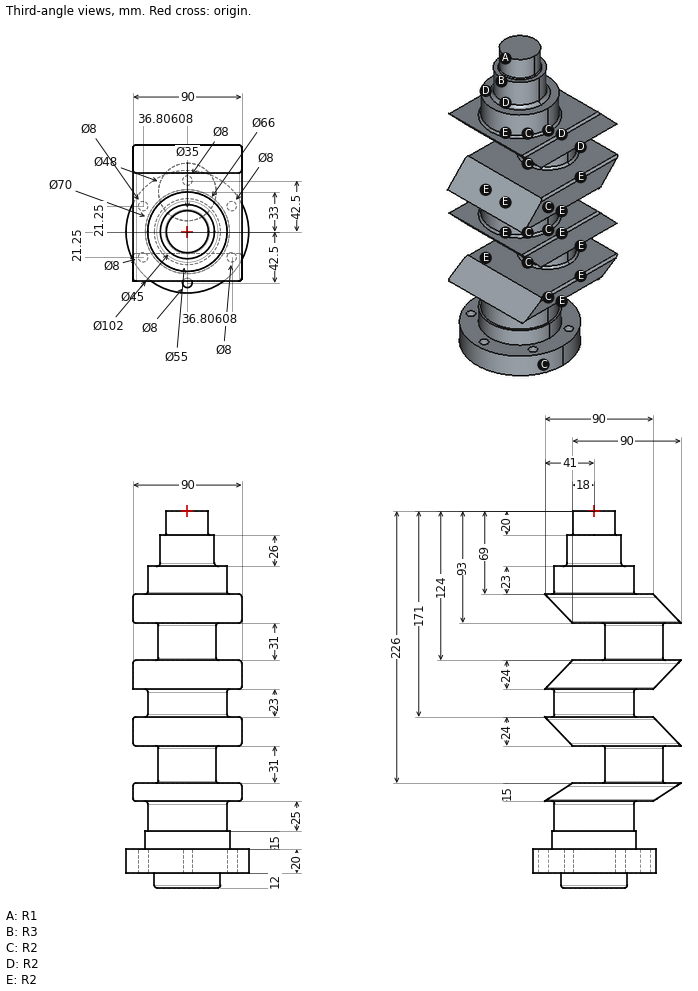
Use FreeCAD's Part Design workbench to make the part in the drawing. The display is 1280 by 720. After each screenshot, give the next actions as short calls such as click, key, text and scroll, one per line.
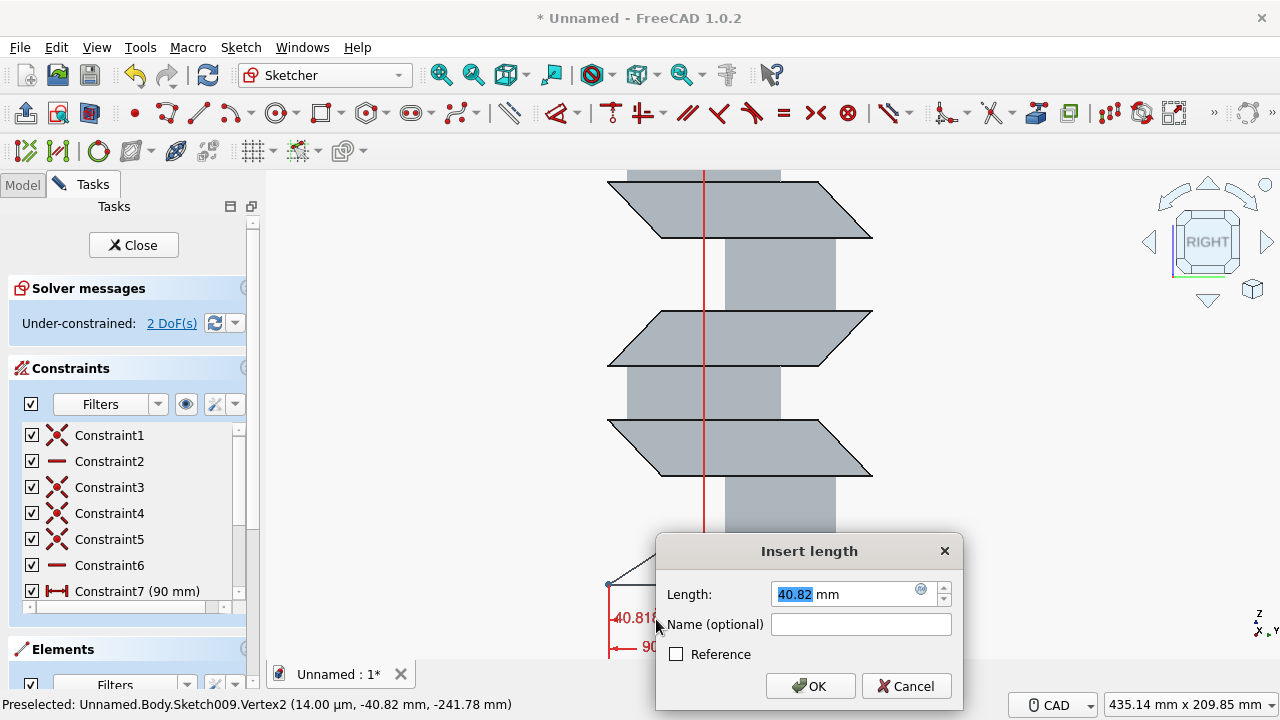
text(41)
key(Return)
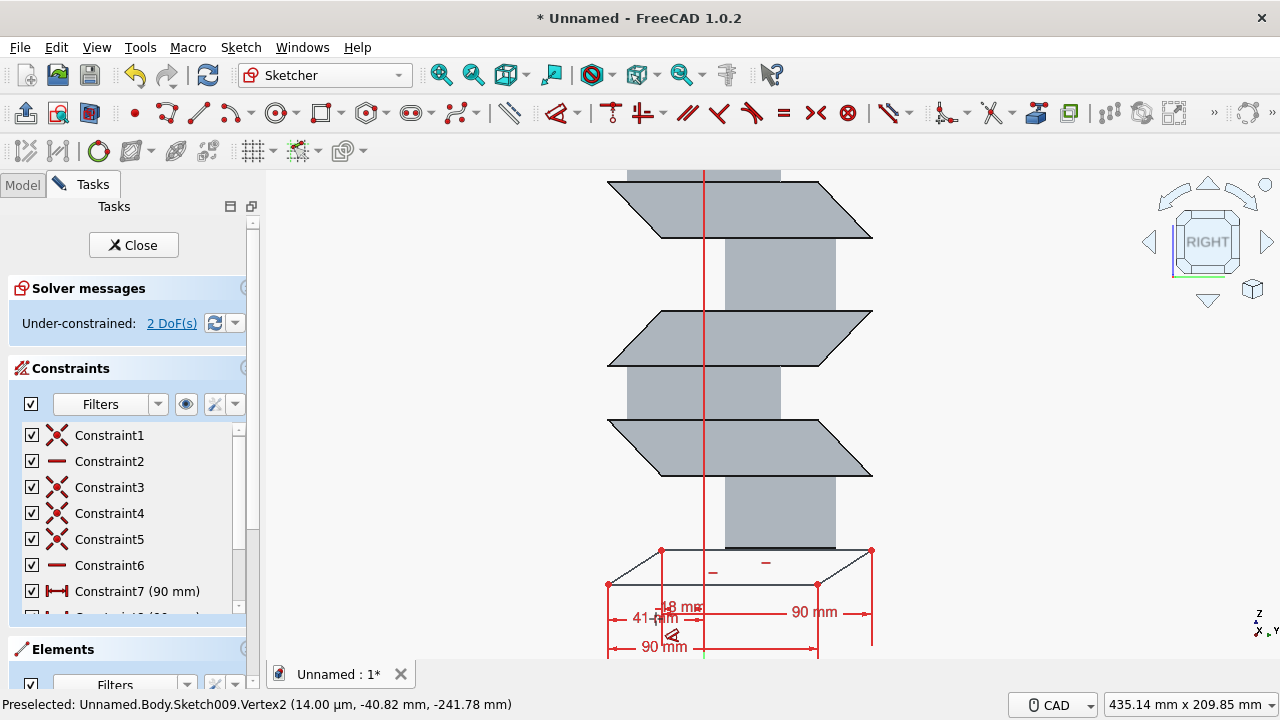
click(646, 561)
click(574, 568)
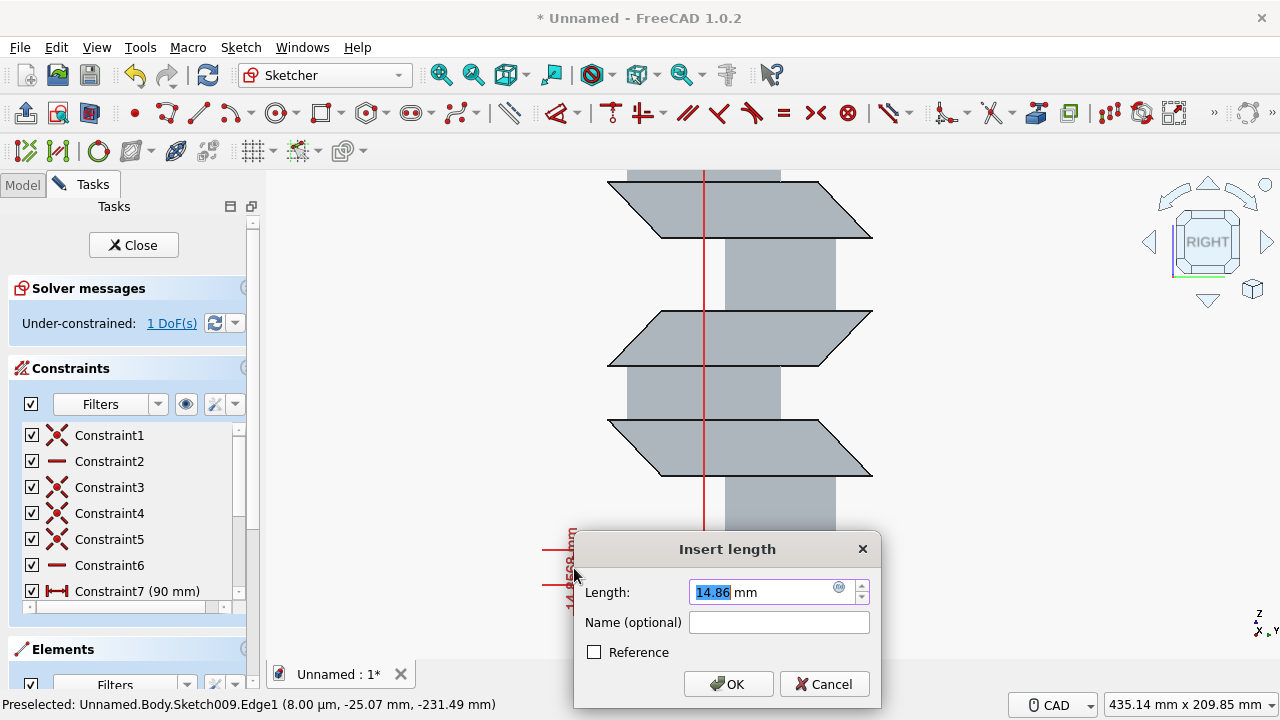
text(15)
key(Return)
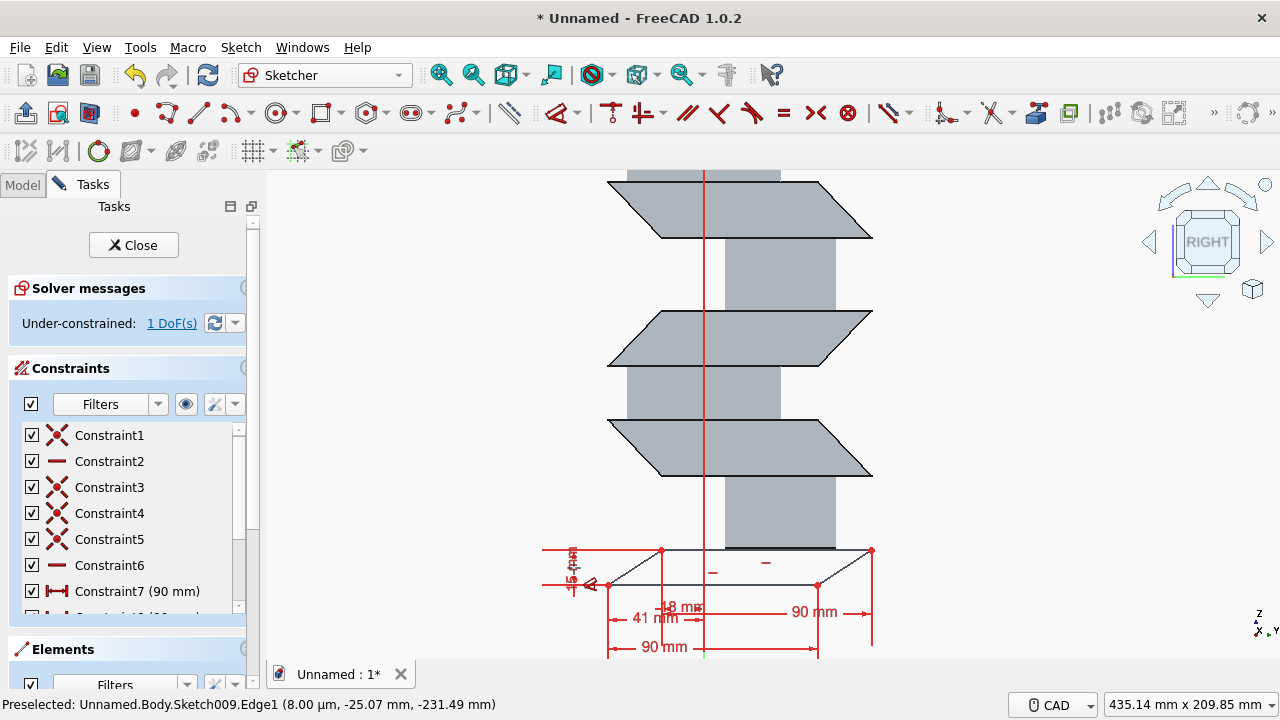
click(662, 550)
click(628, 374)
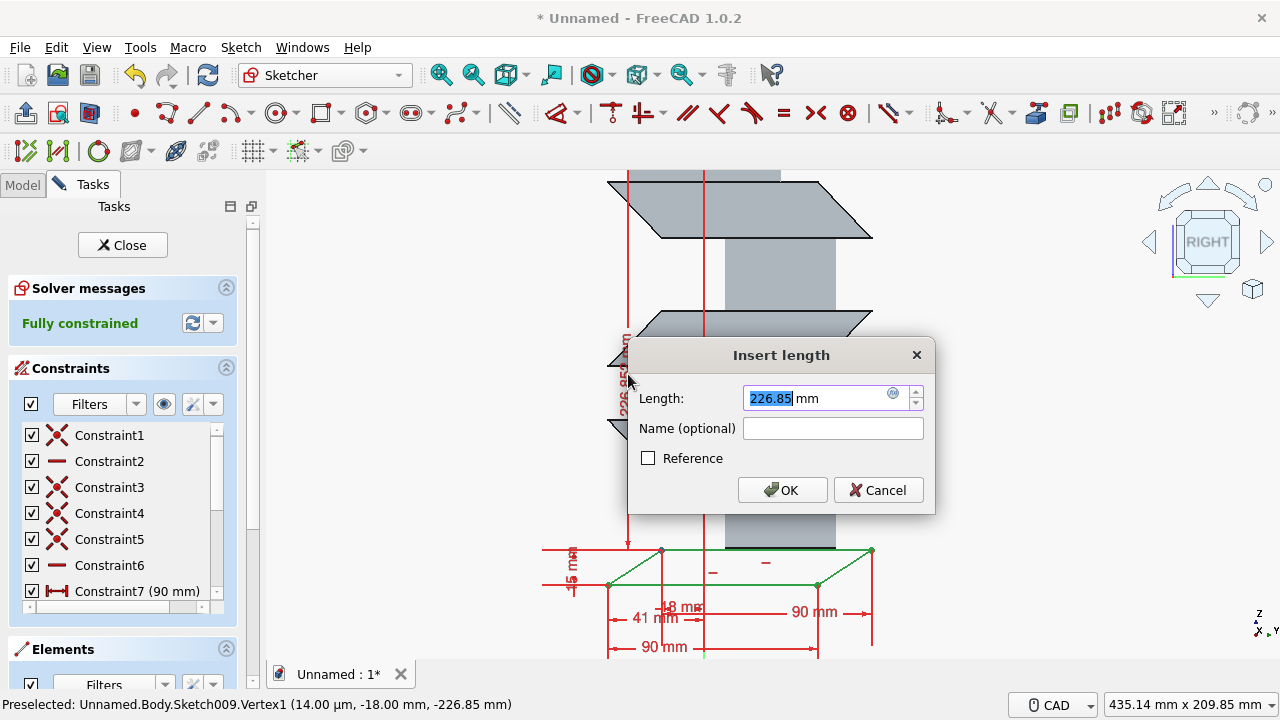
text(226)
key(Return)
key(Escape)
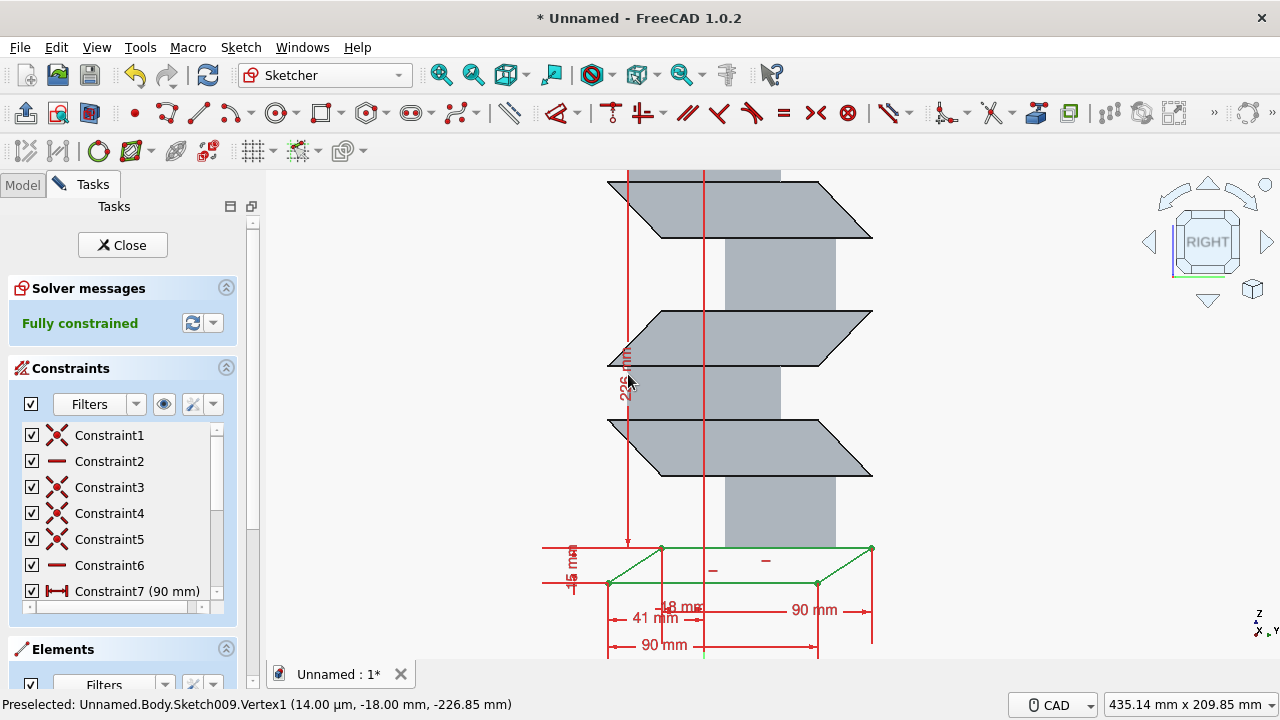
click(123, 245)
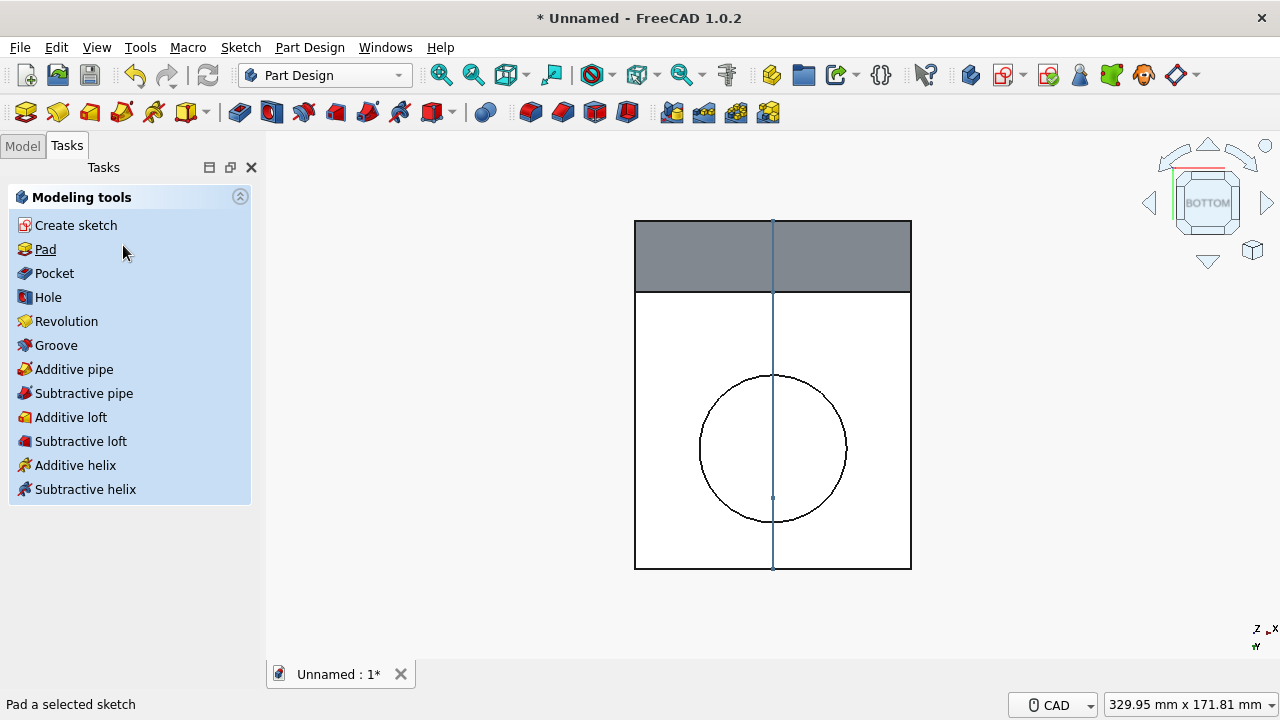
click(26, 112)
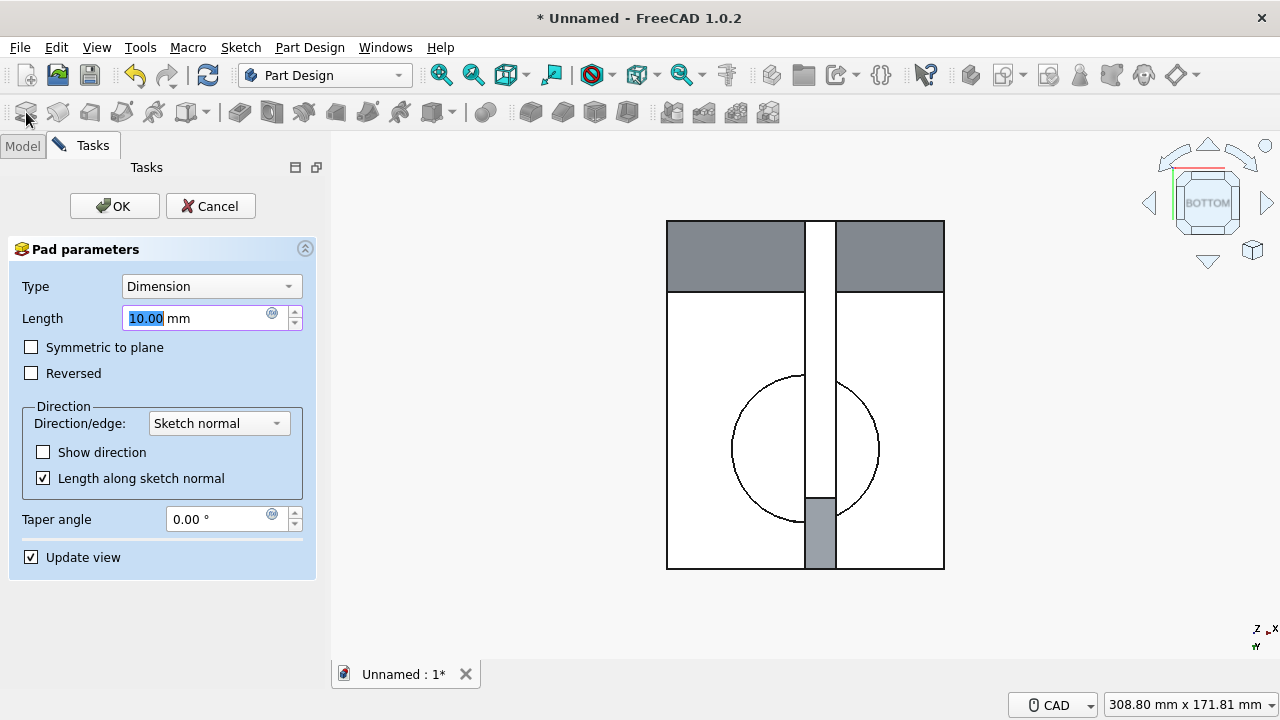
text(90)
key(Tab)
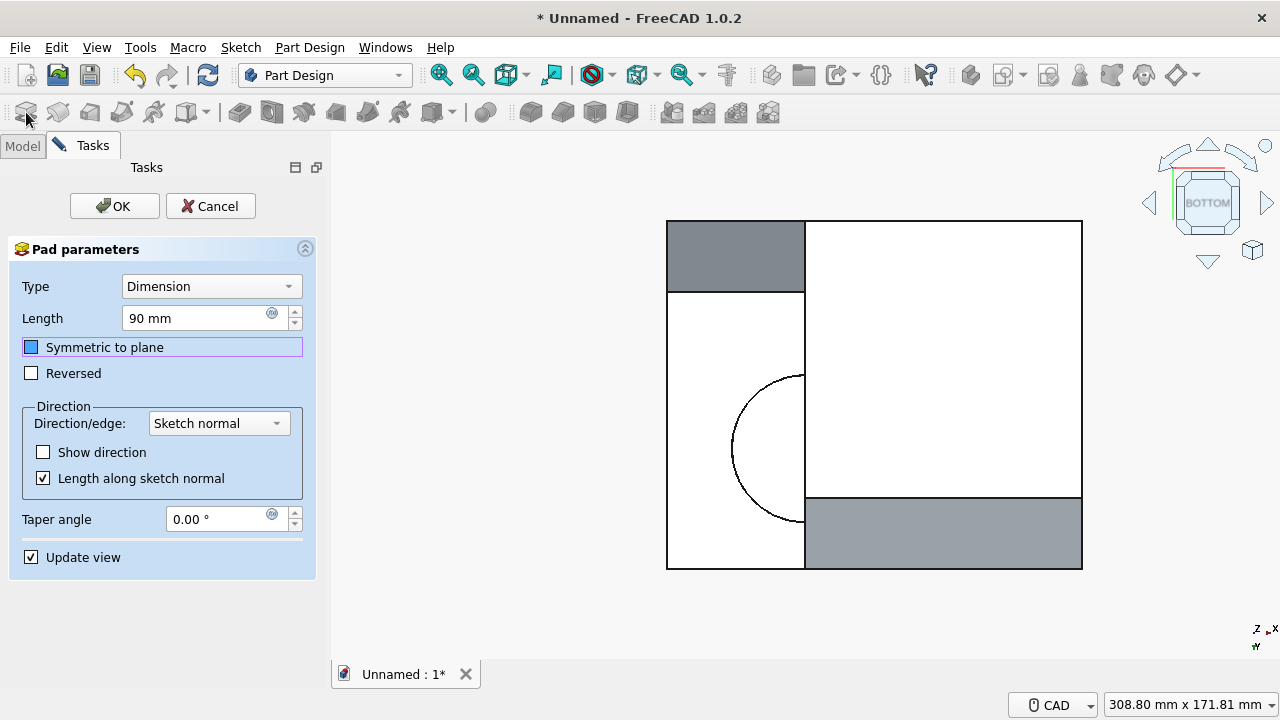
click(30, 347)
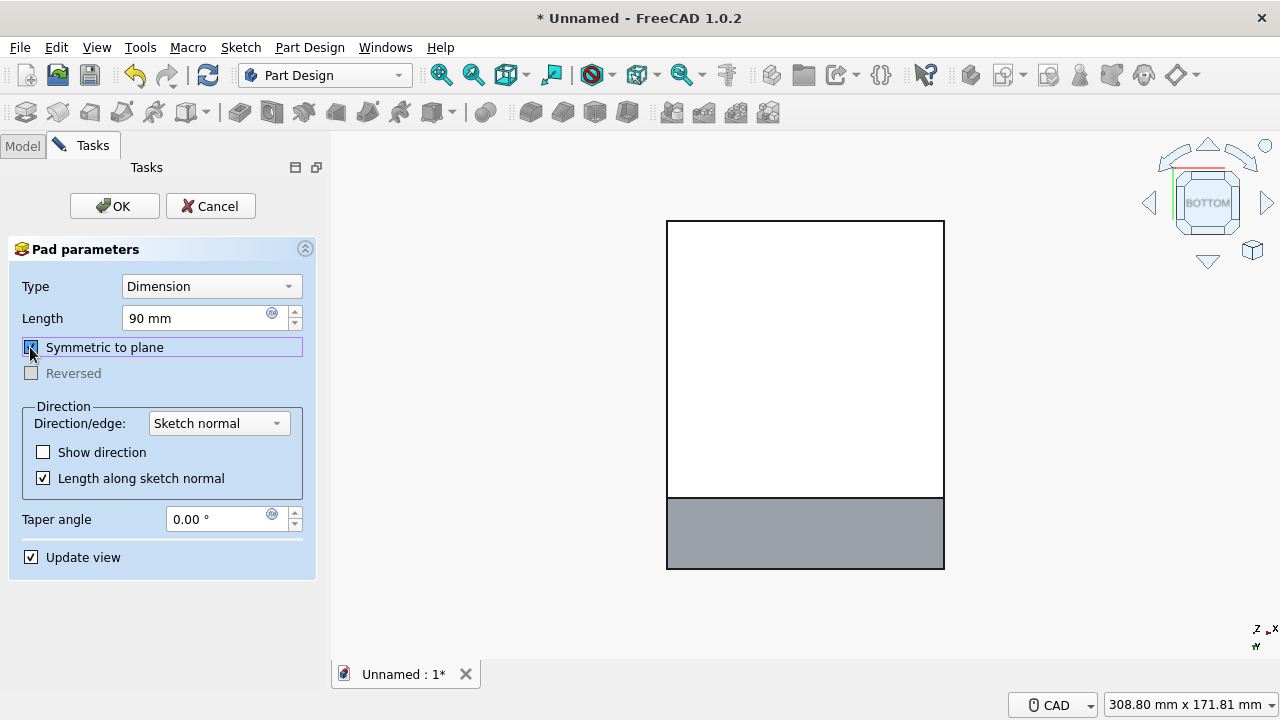
click(115, 206)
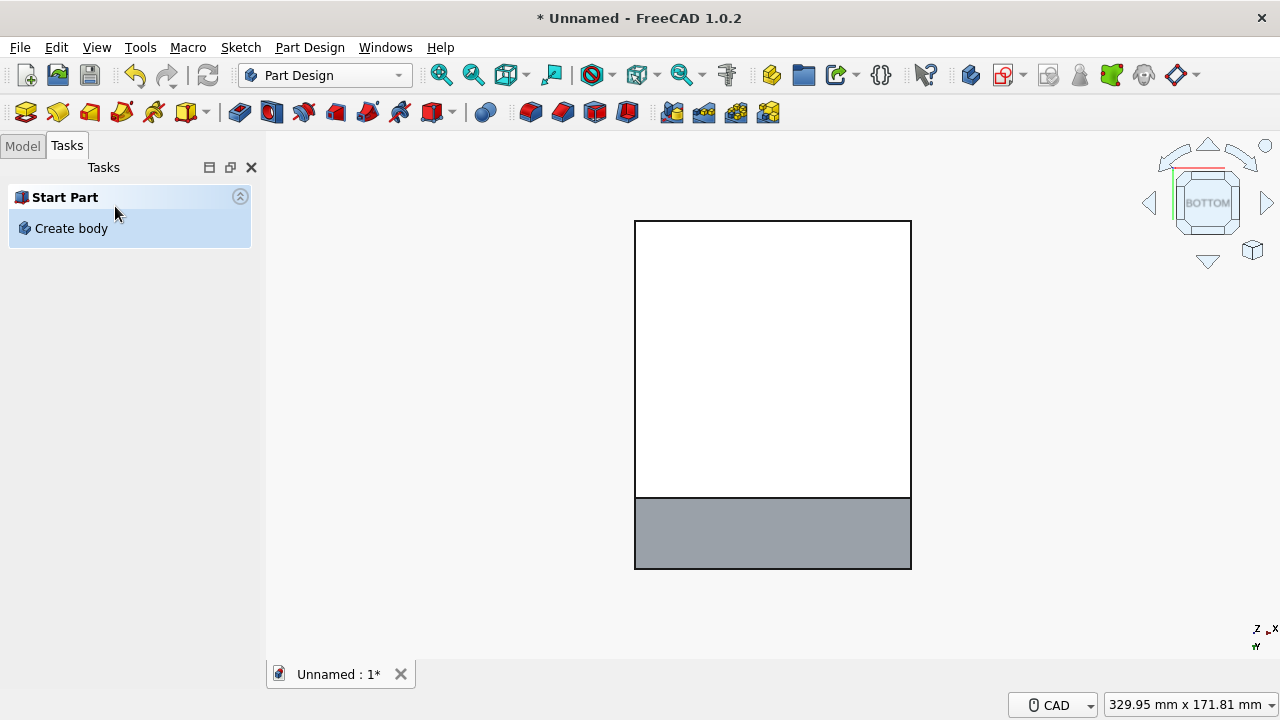
click(773, 359)